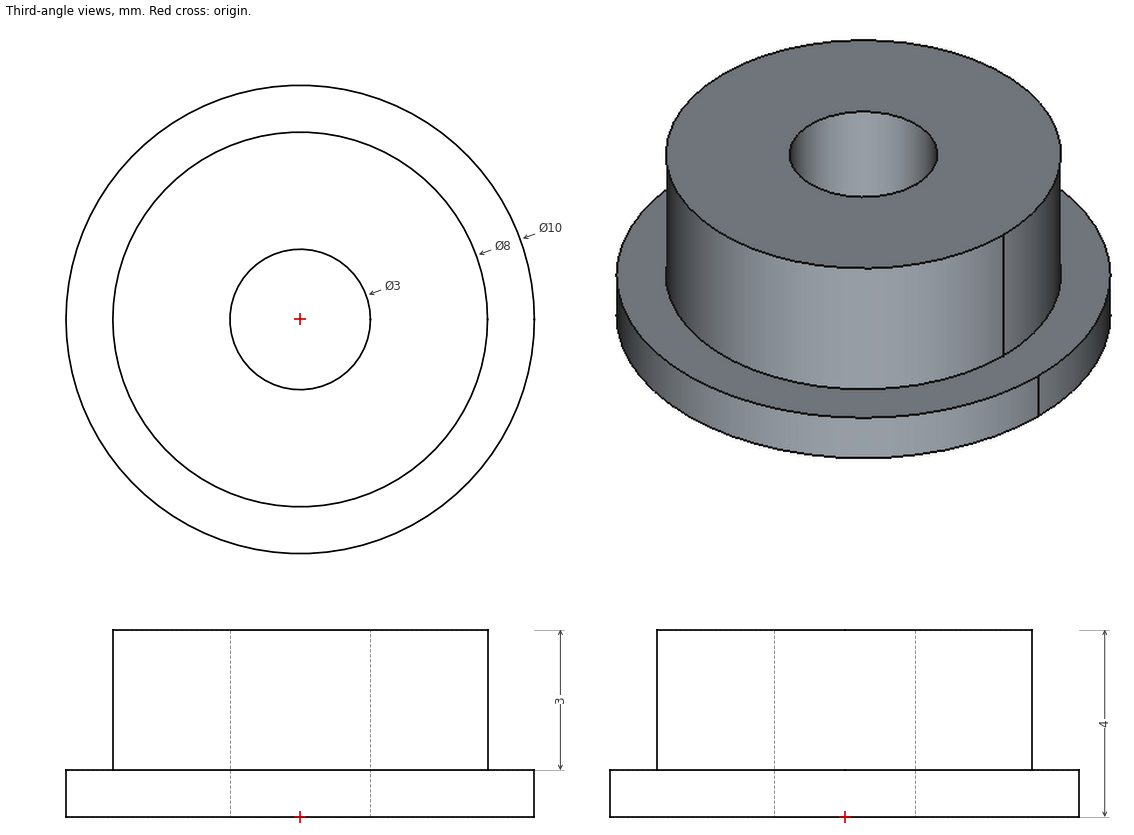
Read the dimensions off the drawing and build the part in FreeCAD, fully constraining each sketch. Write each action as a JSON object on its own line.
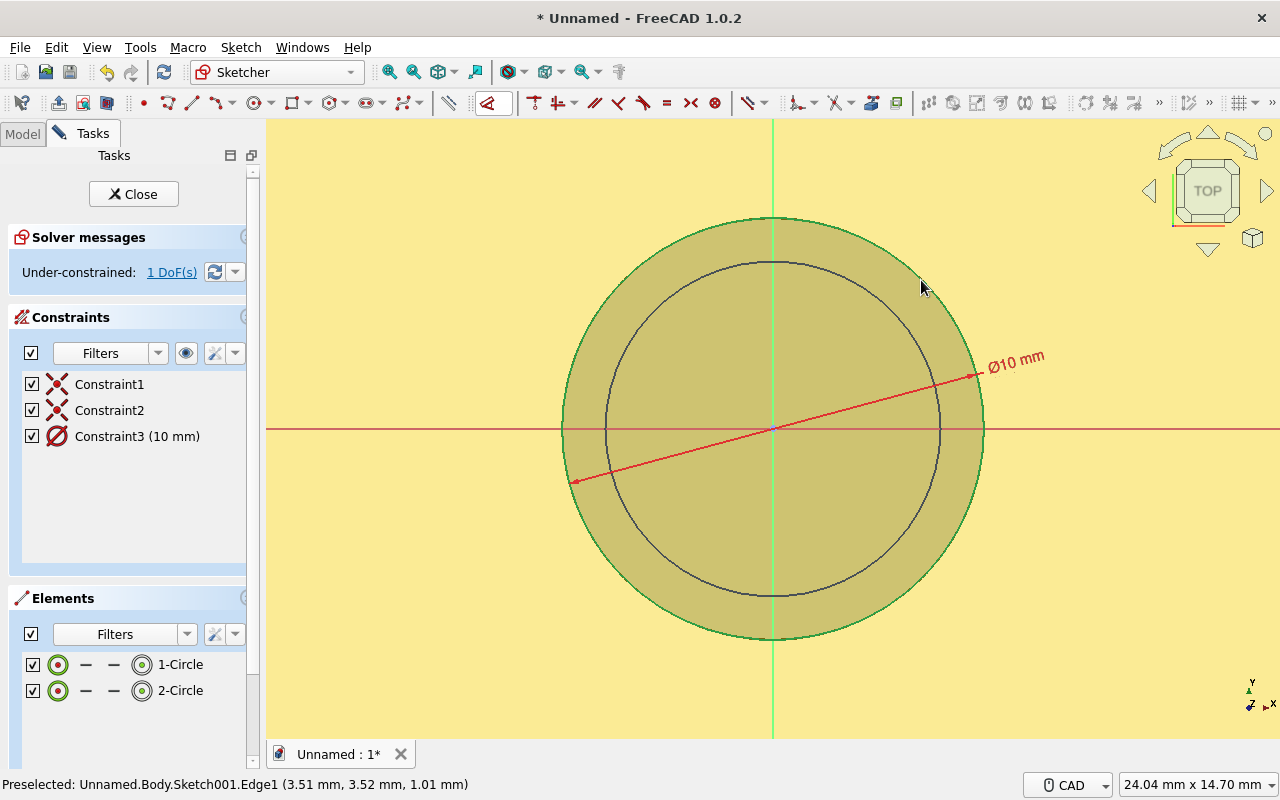
{"action": "left_click", "coordinate": [891, 310]}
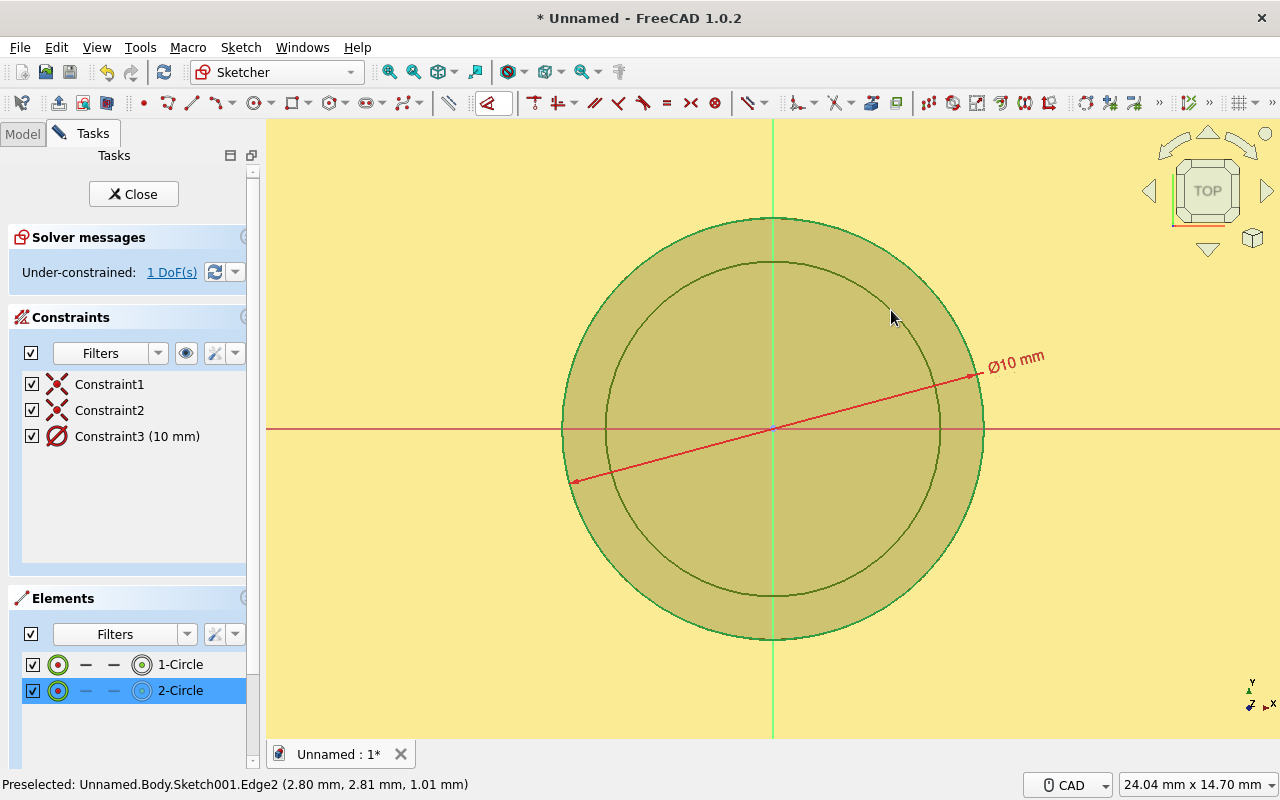
{"action": "key", "text": "k o"}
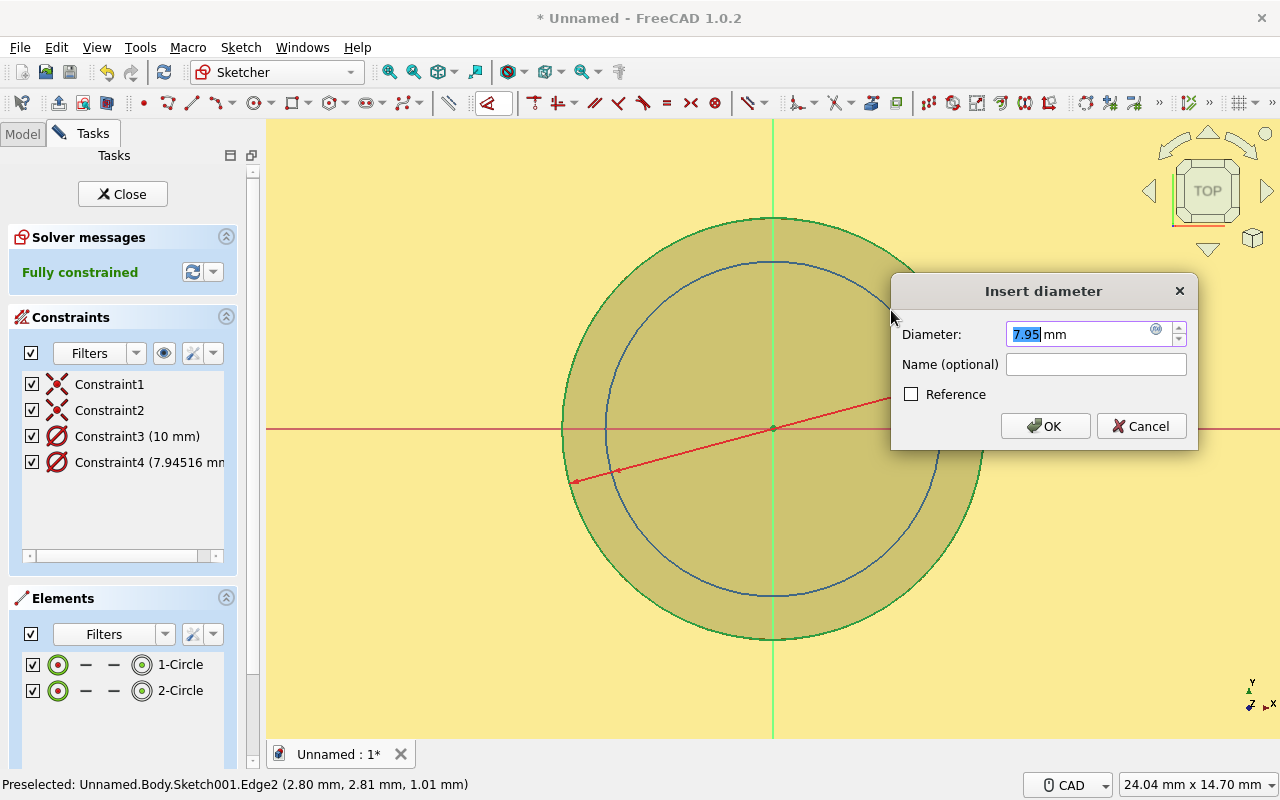
{"action": "type", "text": "8"}
{"action": "key", "text": "Return"}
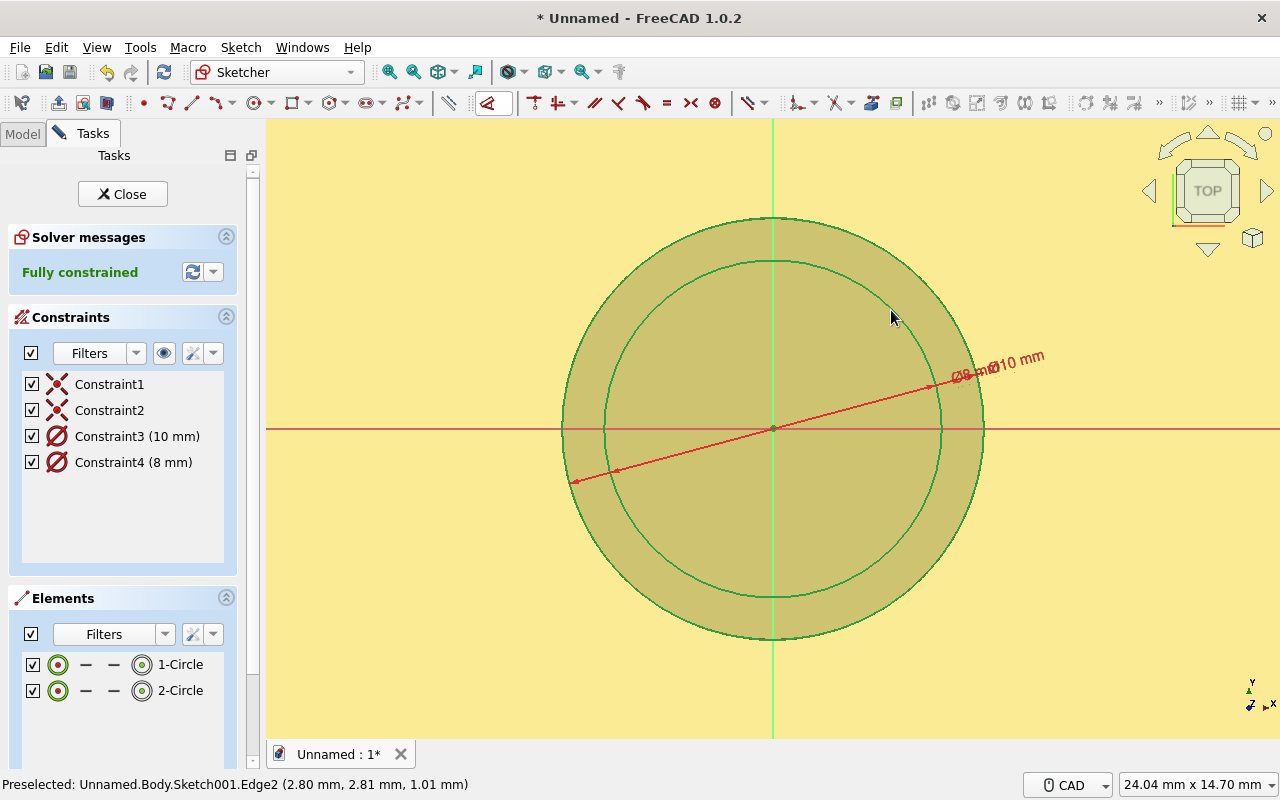
{"action": "left_click", "coordinate": [123, 194]}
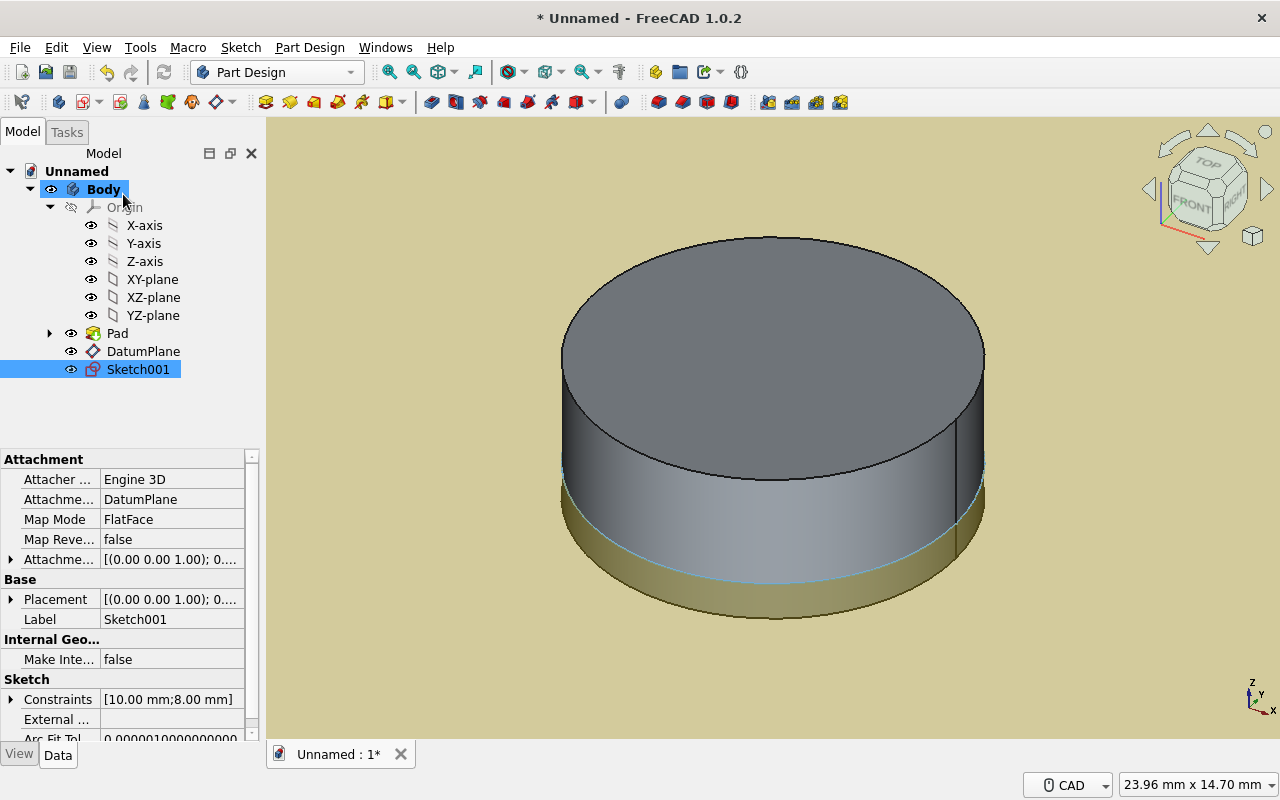
{"action": "left_click", "coordinate": [432, 102]}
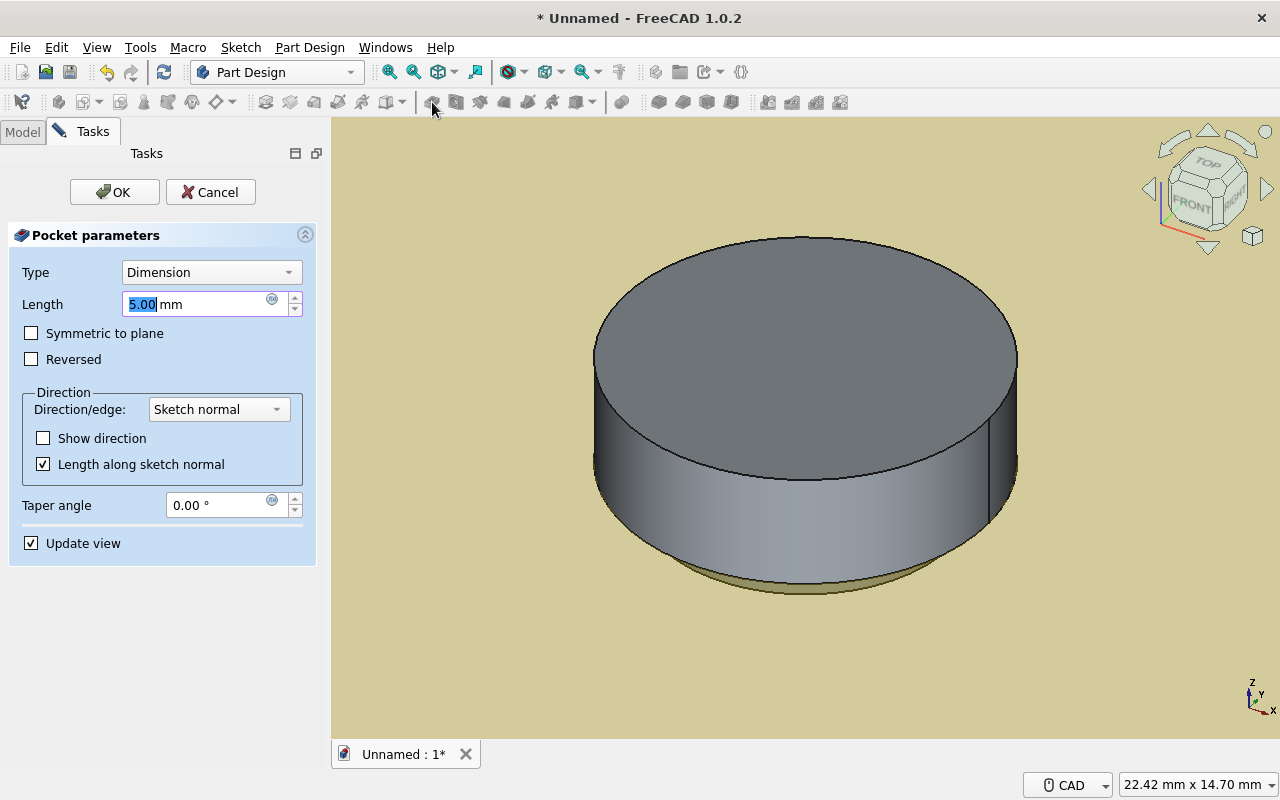
{"action": "type", "text": "3"}
{"action": "key", "text": "Tab"}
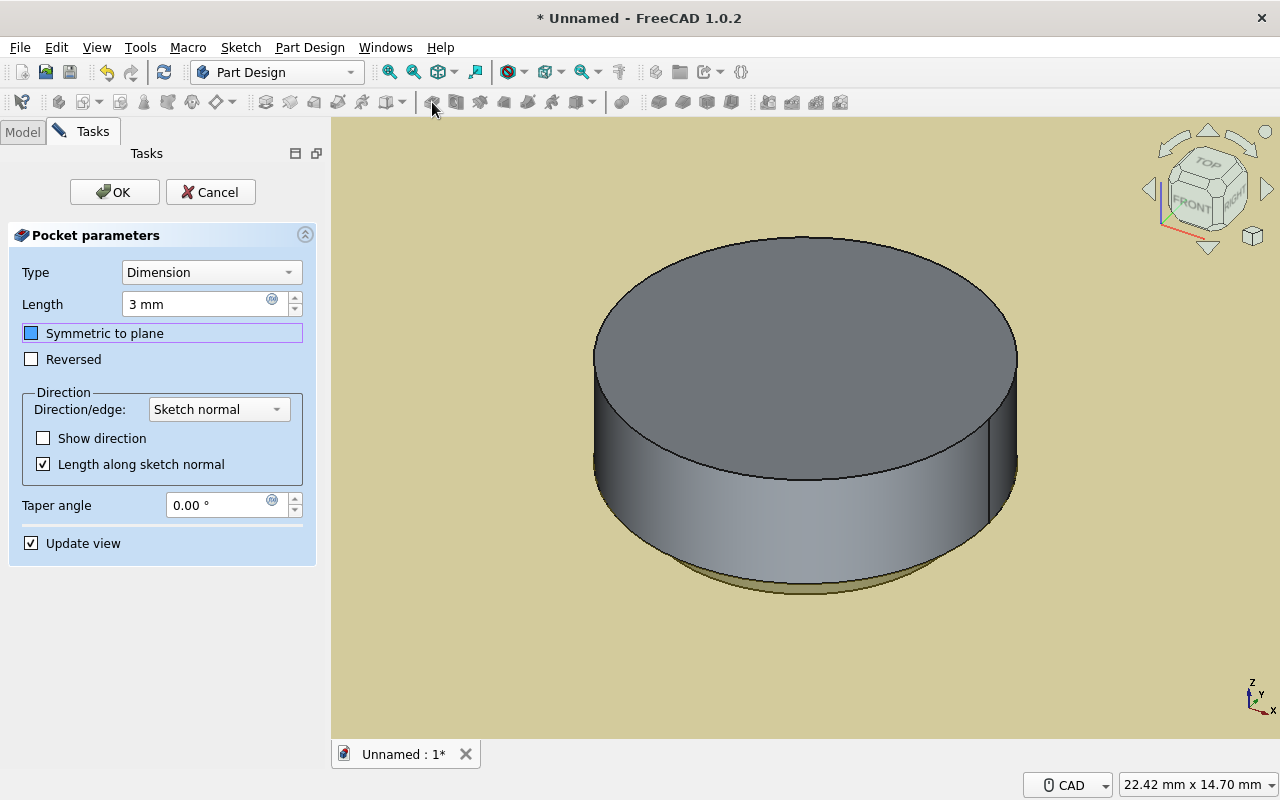
{"action": "left_click", "coordinate": [30, 359]}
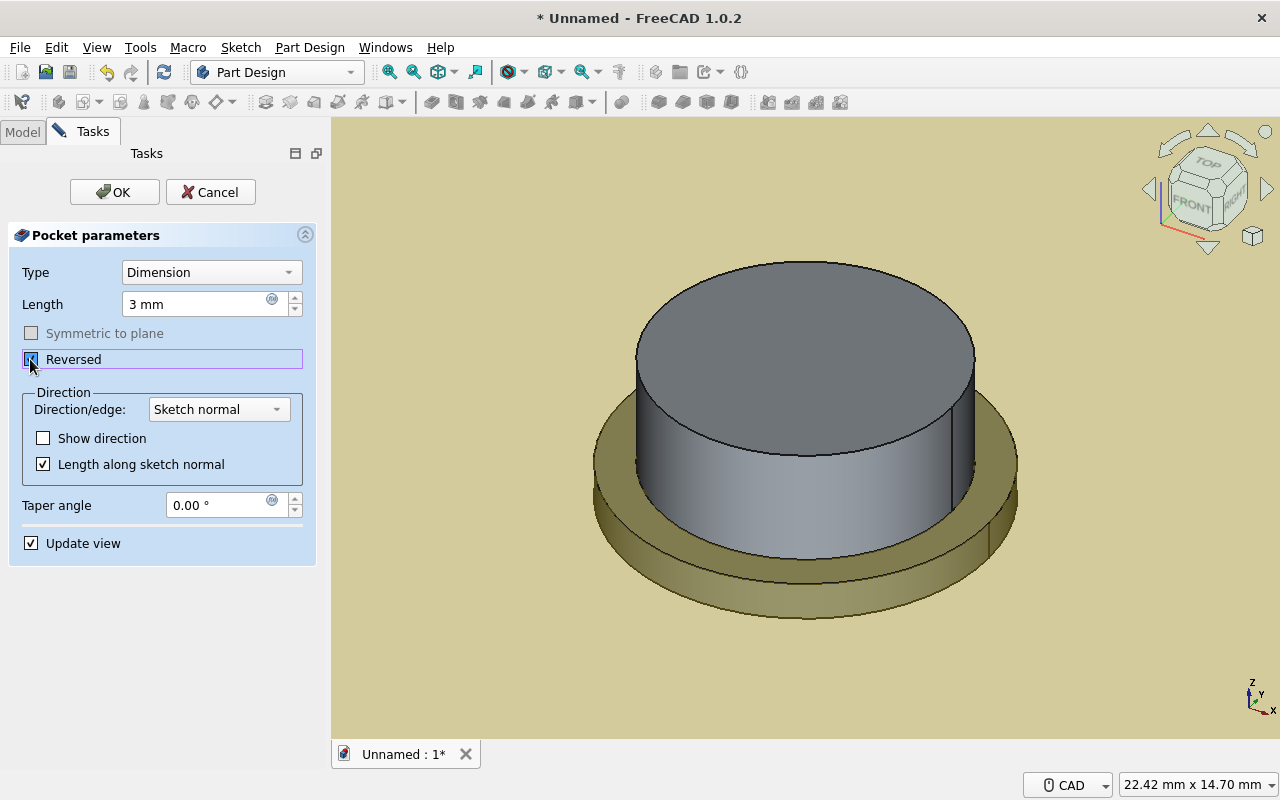
{"action": "left_click", "coordinate": [115, 192]}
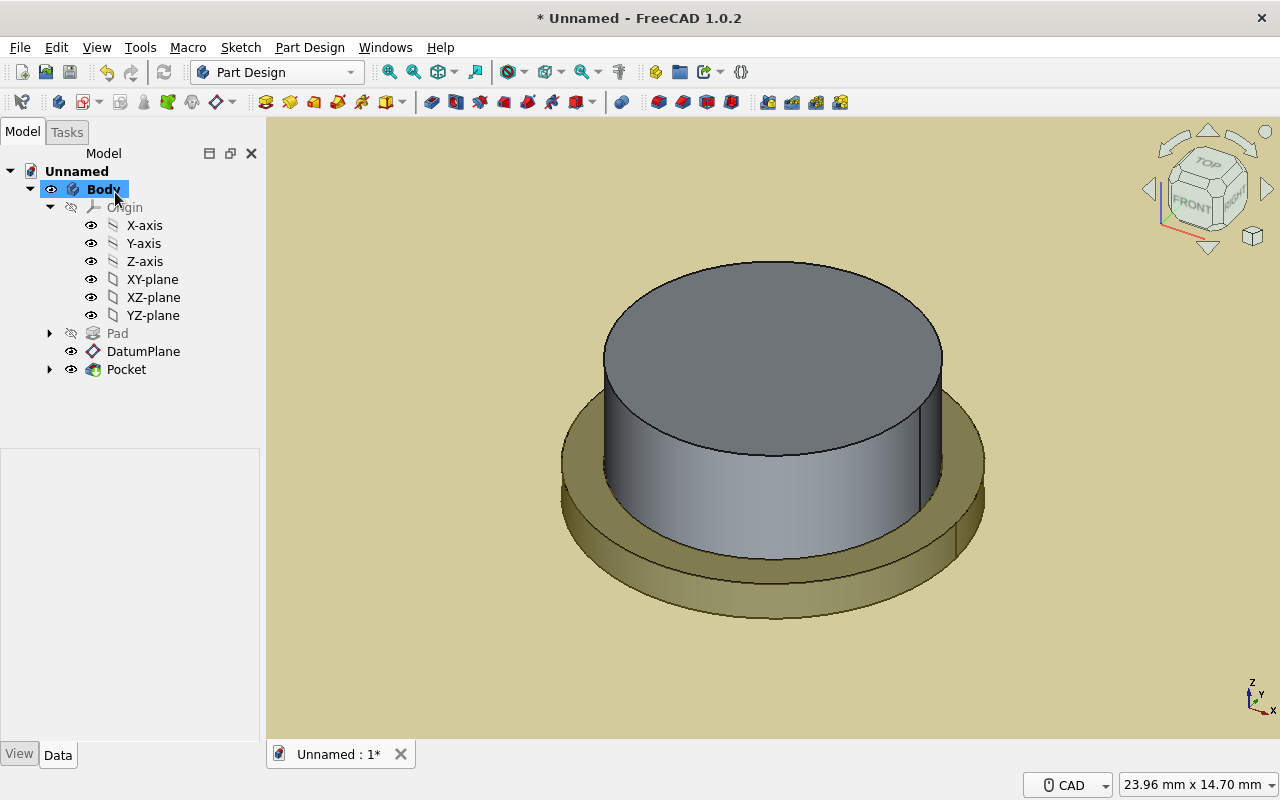
{"action": "left_click", "coordinate": [116, 351]}
{"action": "key", "text": "space"}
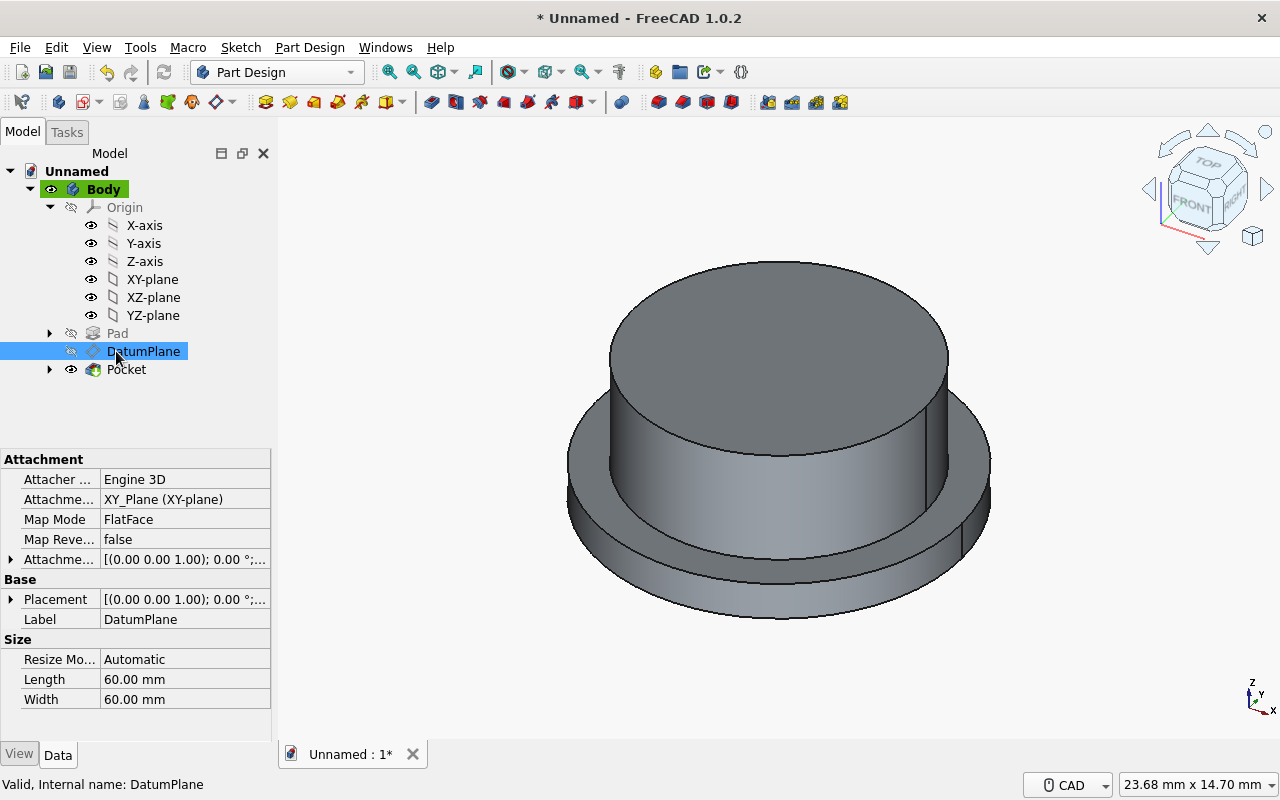
{"action": "left_click", "coordinate": [779, 358]}